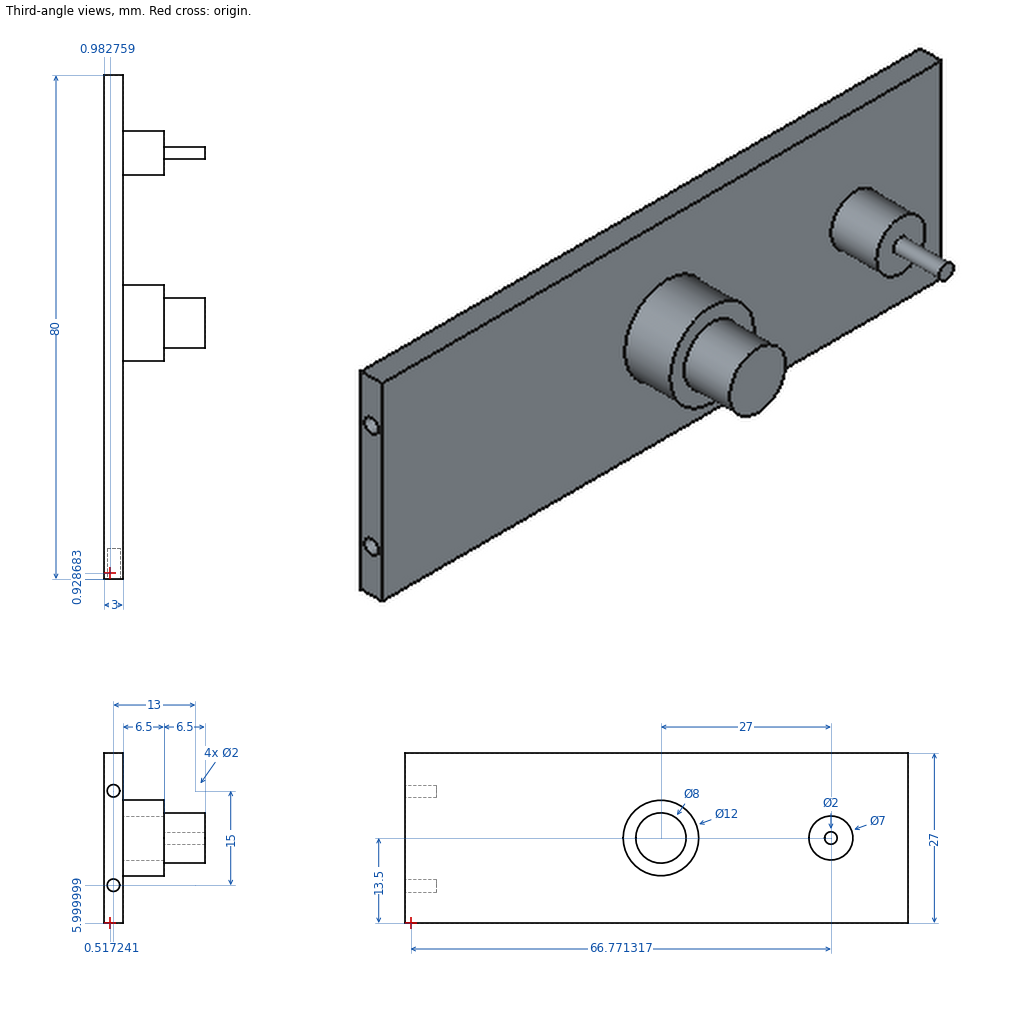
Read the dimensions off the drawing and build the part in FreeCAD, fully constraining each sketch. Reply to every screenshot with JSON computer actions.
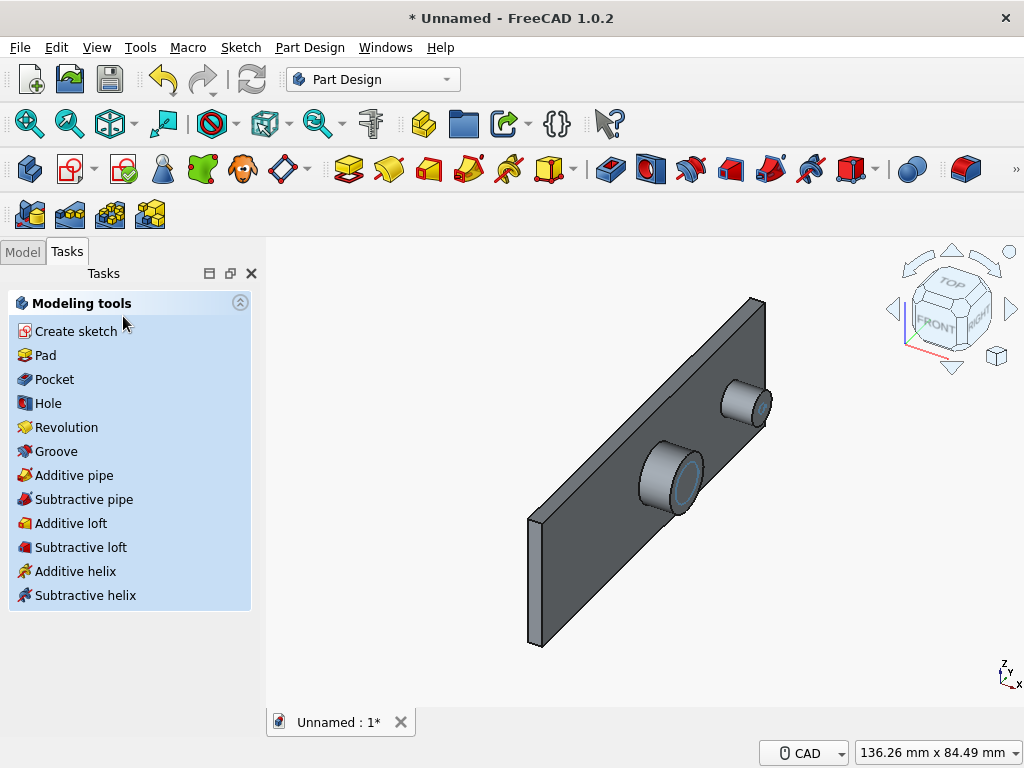
{"action": "left_click", "coordinate": [350, 170]}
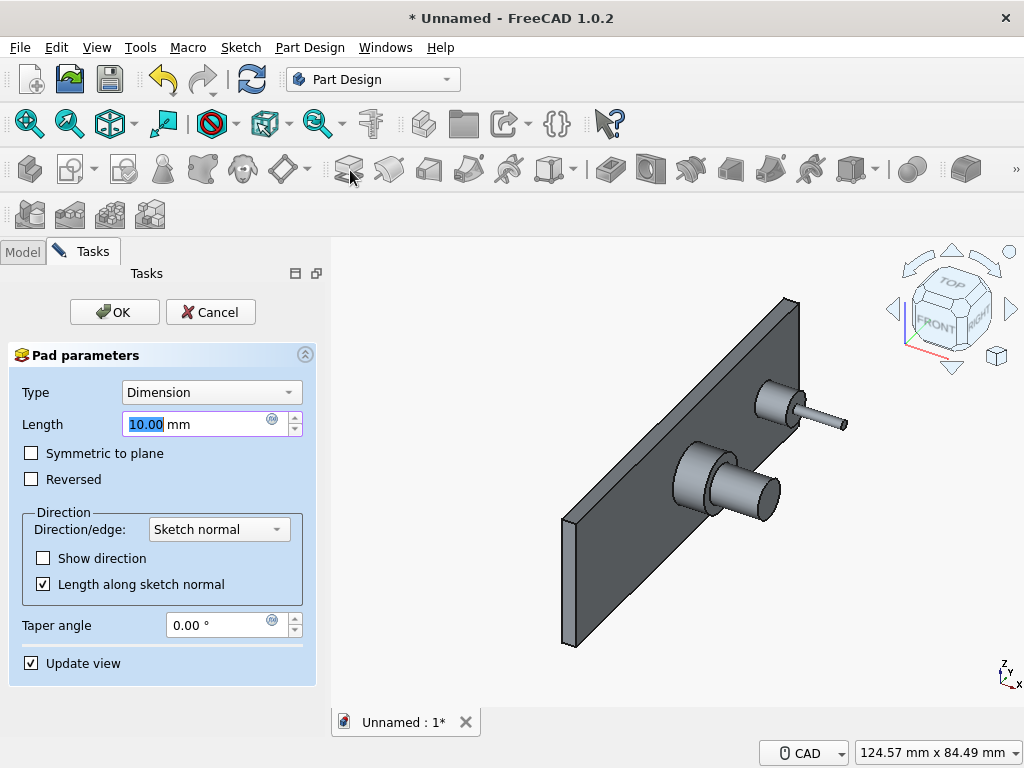
{"action": "type", "text": "6.5"}
{"action": "key", "text": "Tab"}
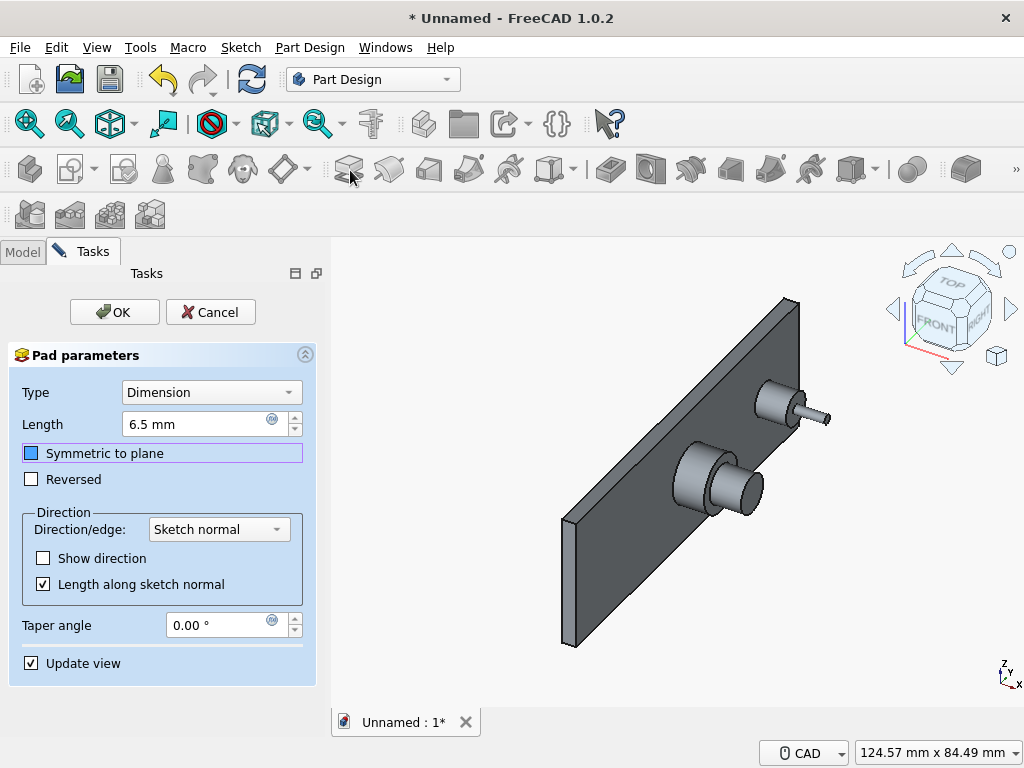
{"action": "left_click", "coordinate": [115, 312]}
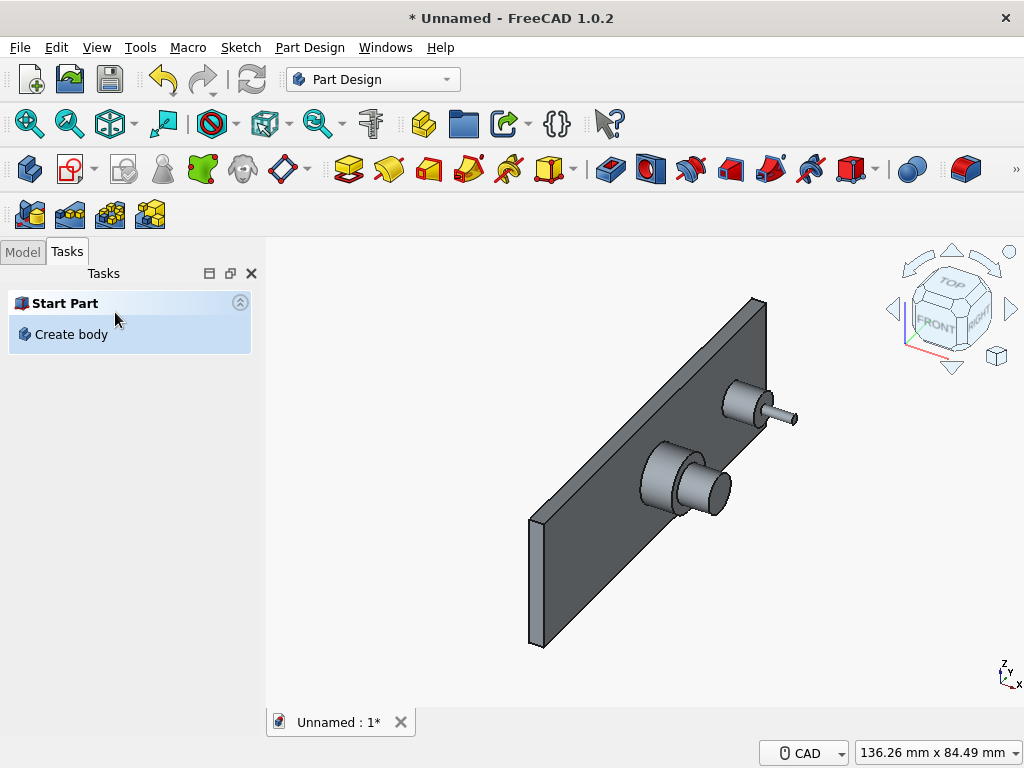
{"action": "left_click", "coordinate": [23, 251]}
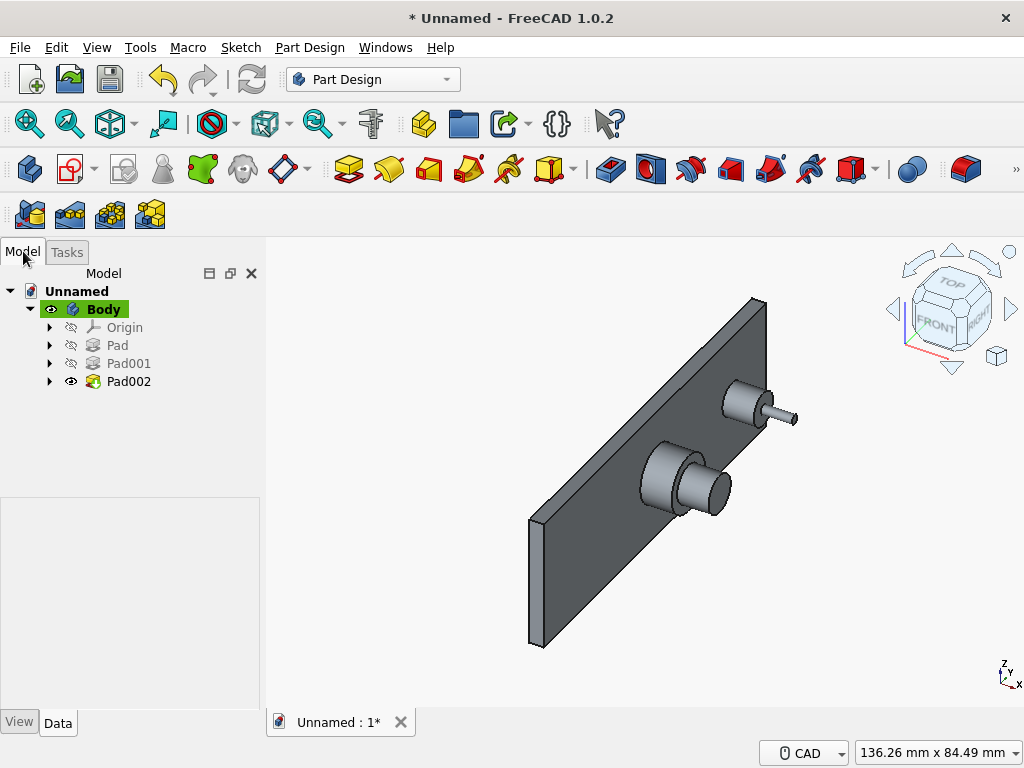
{"action": "left_click", "coordinate": [50, 327]}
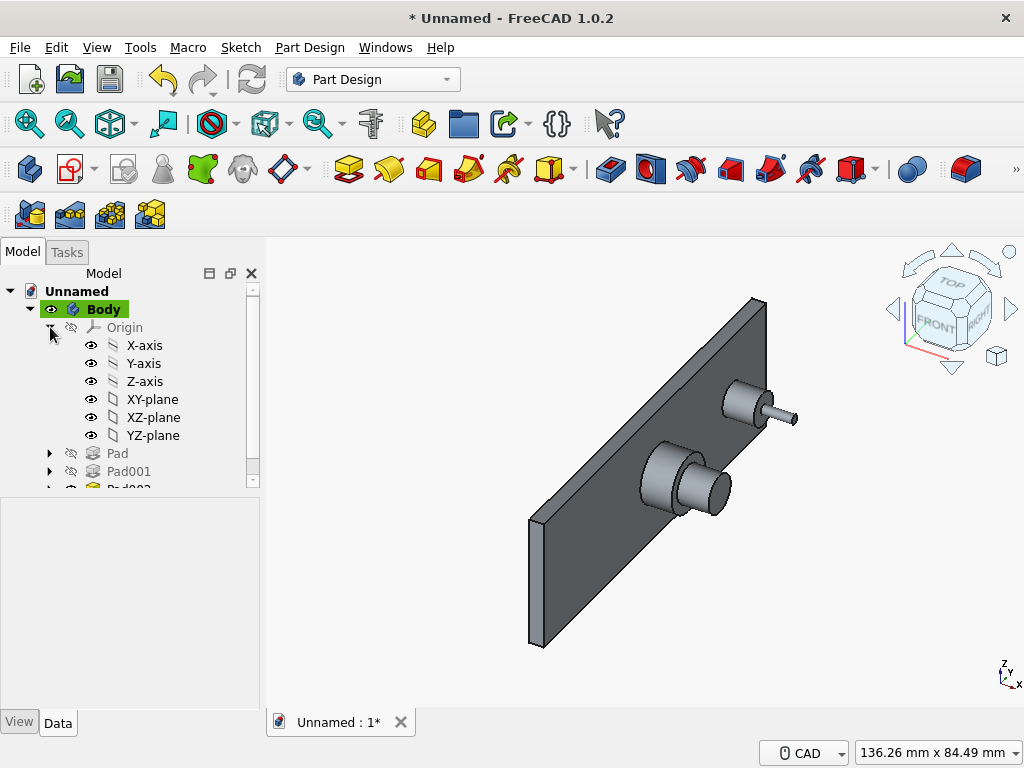
{"action": "left_click", "coordinate": [136, 417]}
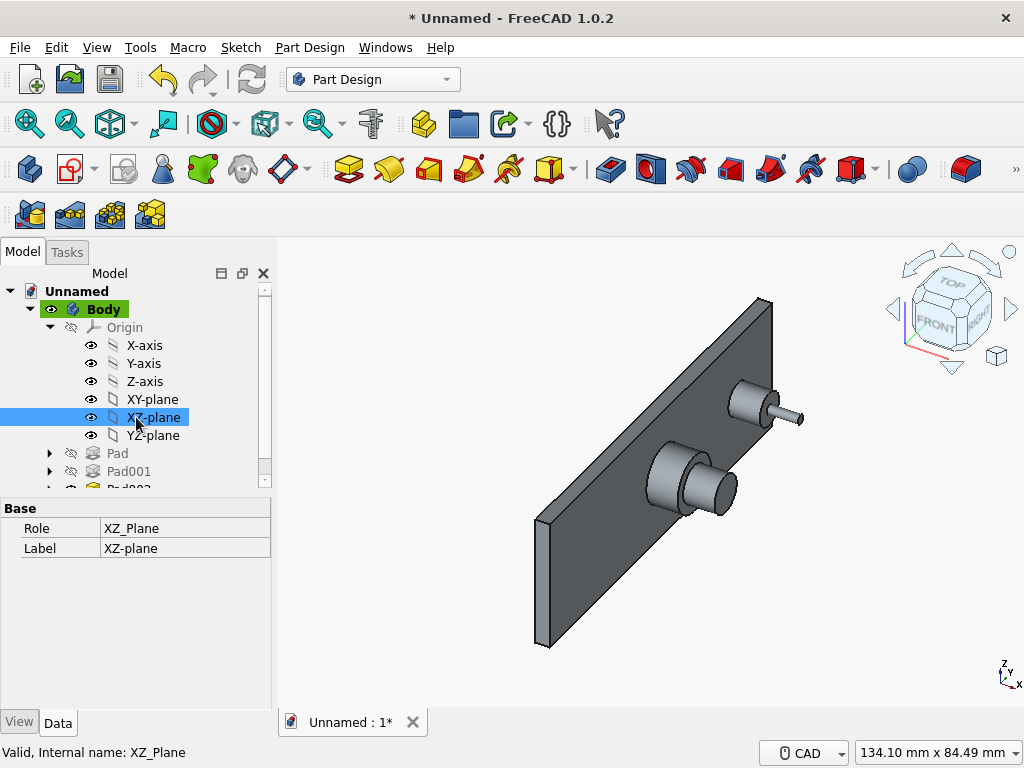
{"action": "left_click", "coordinate": [284, 170]}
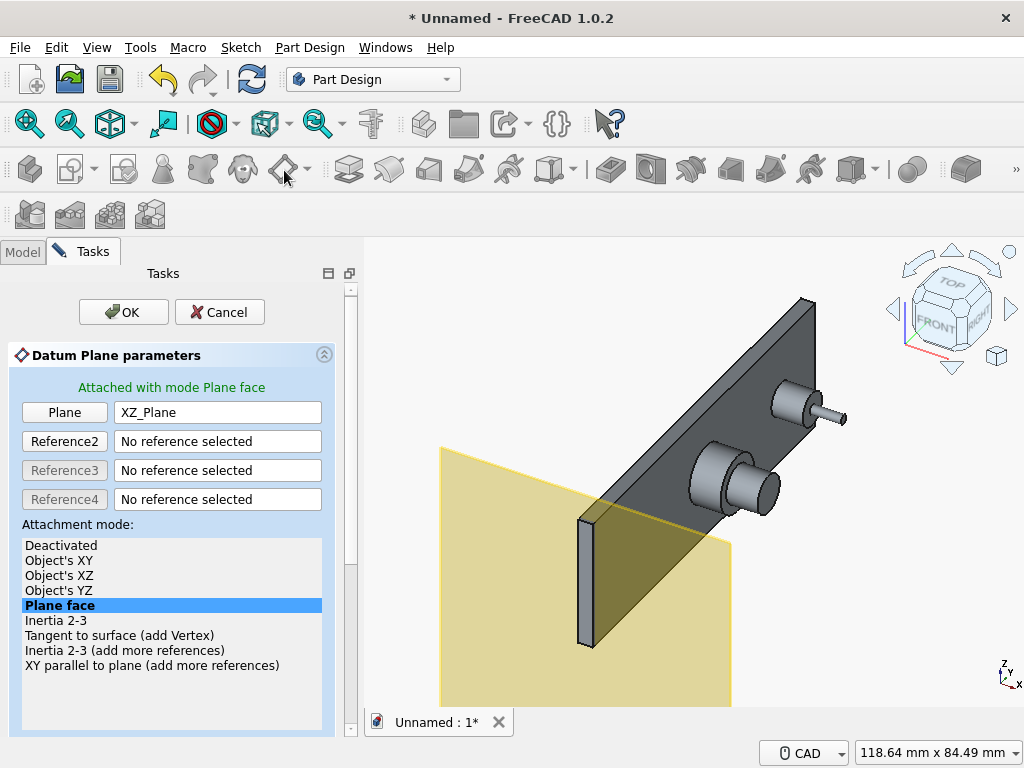
{"action": "scroll", "coordinate": [351, 510], "scroll_direction": "down", "scroll_amount": 3}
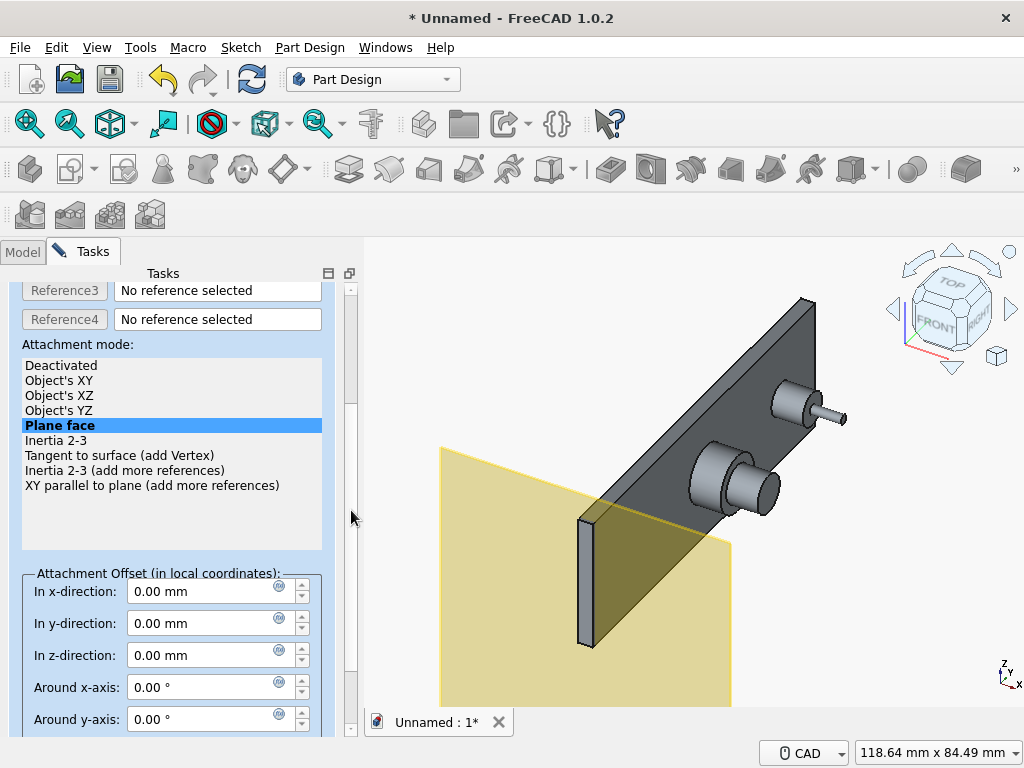
{"action": "triple_click", "coordinate": [210, 655]}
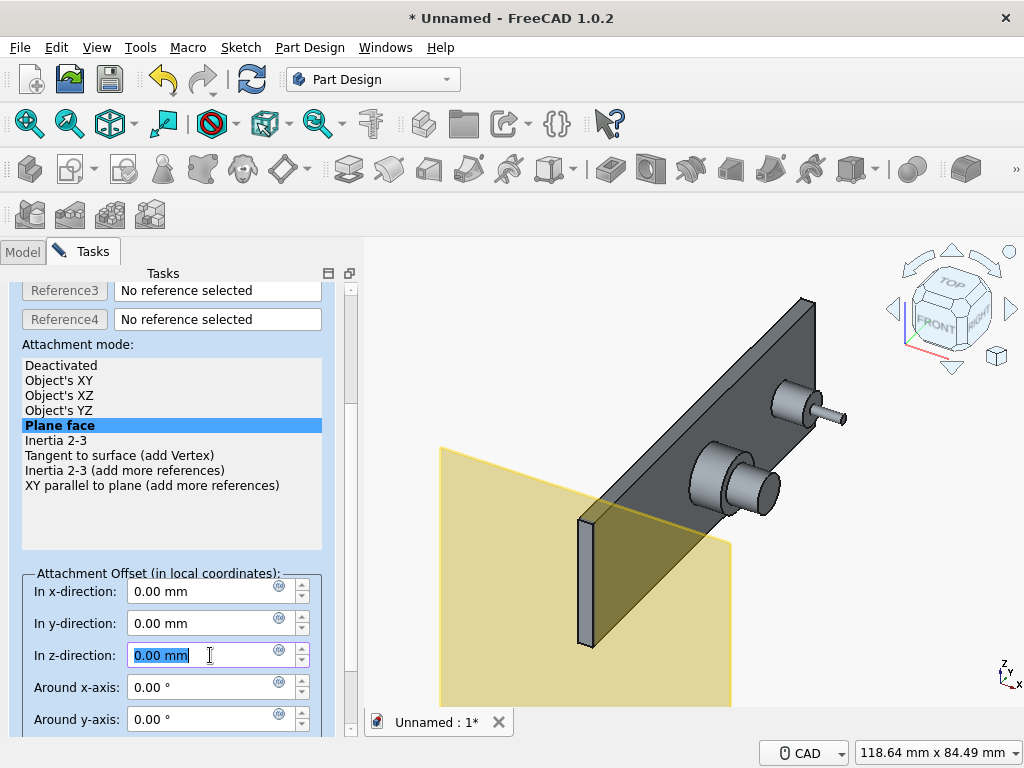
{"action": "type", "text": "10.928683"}
{"action": "key", "text": "Tab"}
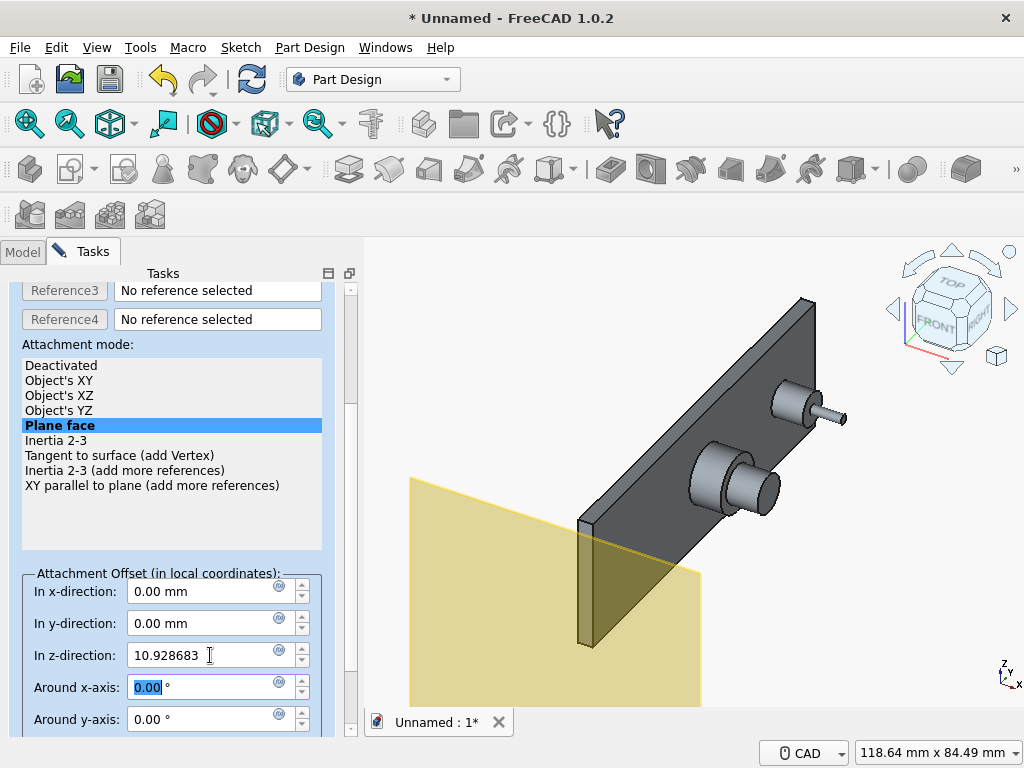
{"action": "scroll", "coordinate": [351, 510], "scroll_direction": "up", "scroll_amount": 4}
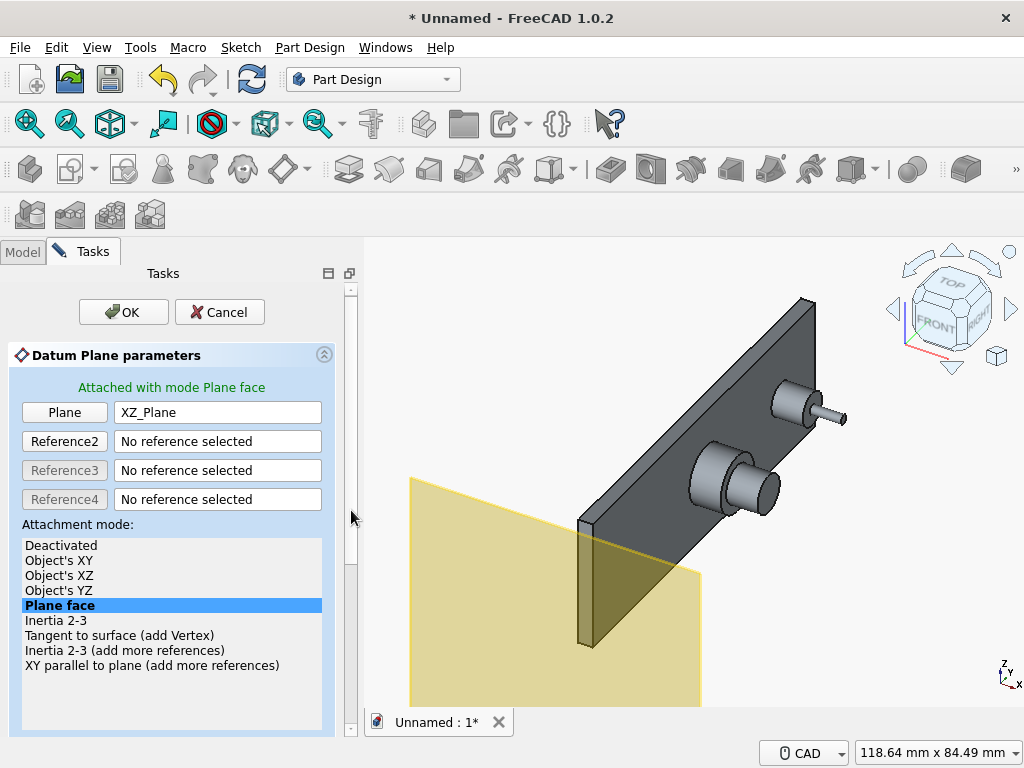
{"action": "left_click", "coordinate": [124, 312]}